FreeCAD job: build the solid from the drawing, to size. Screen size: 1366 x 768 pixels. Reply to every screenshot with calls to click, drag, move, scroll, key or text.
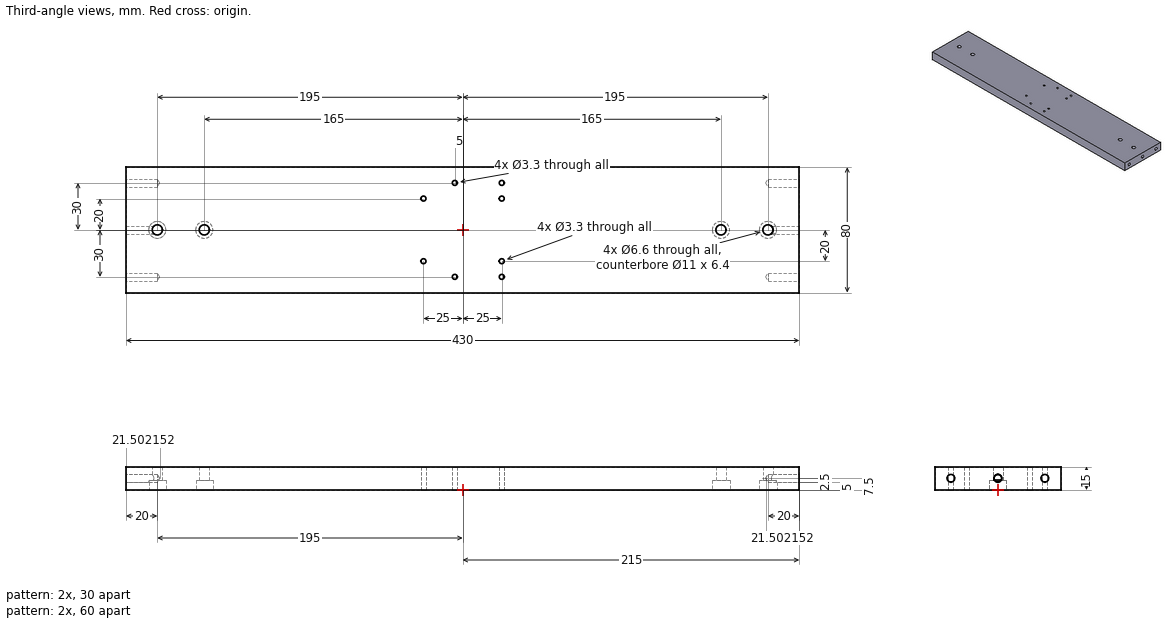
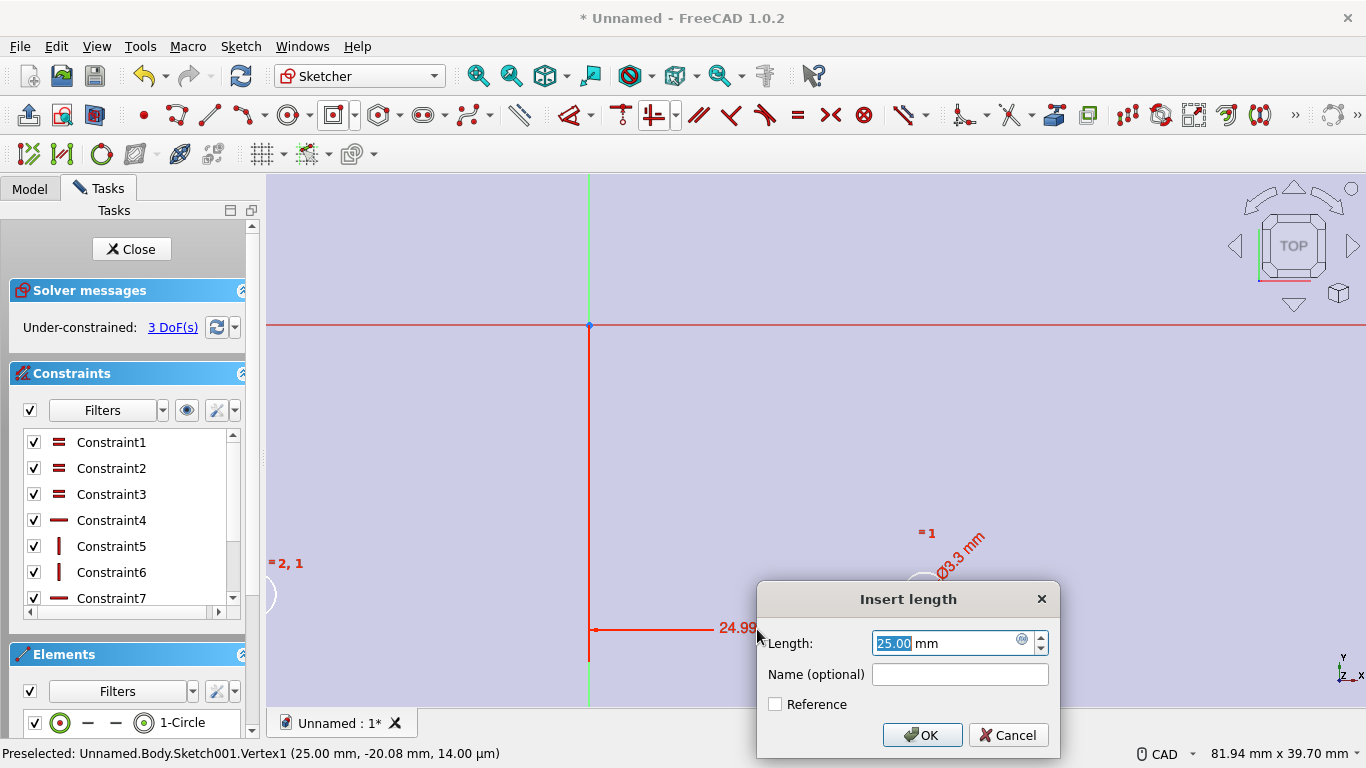
text(25)
key(Return)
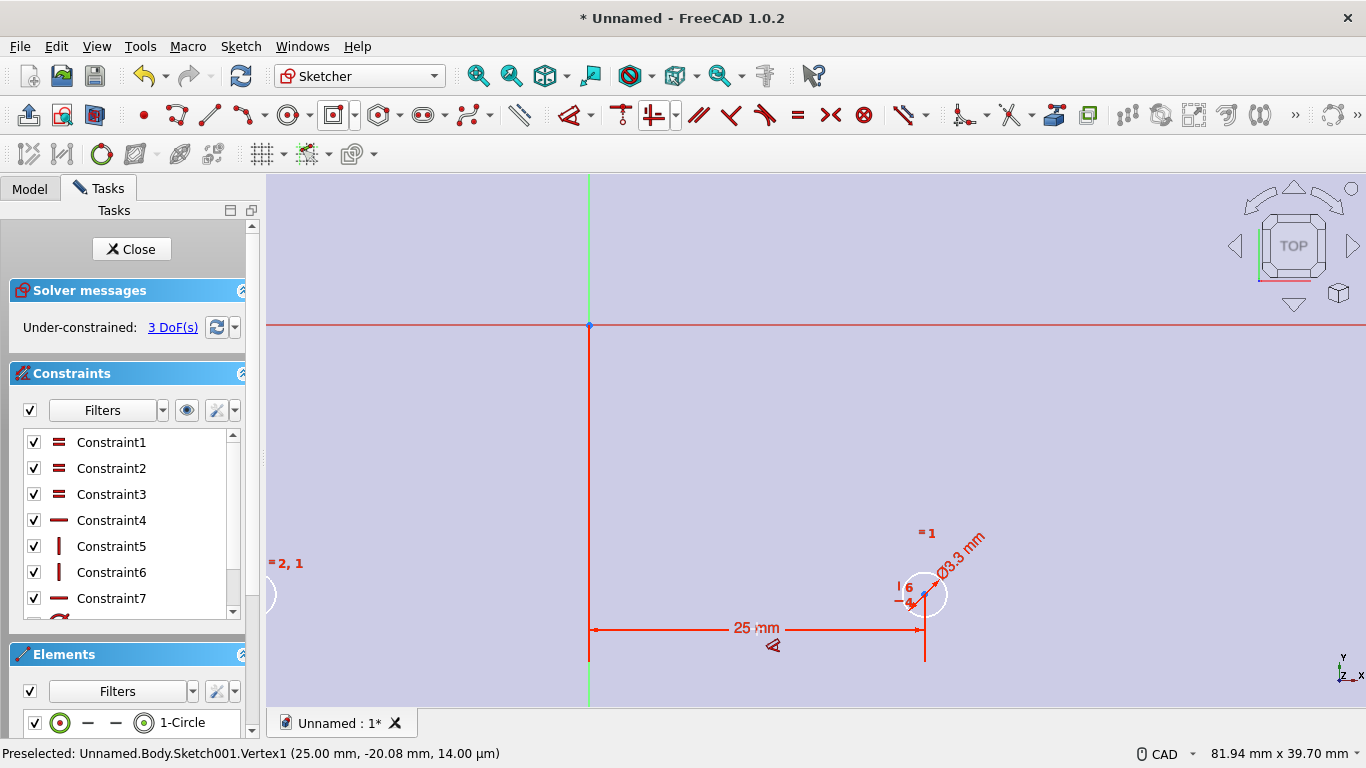
click(925, 595)
click(959, 460)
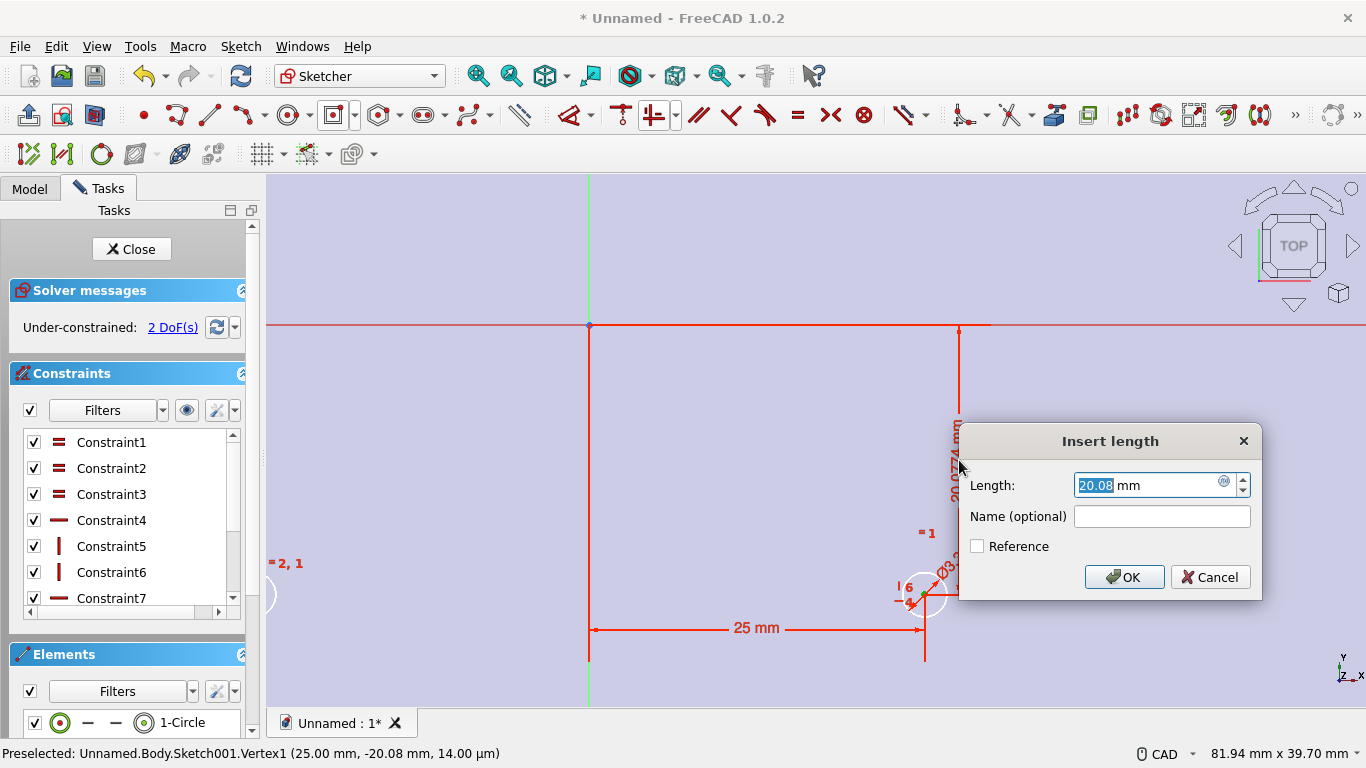
text(20)
key(Return)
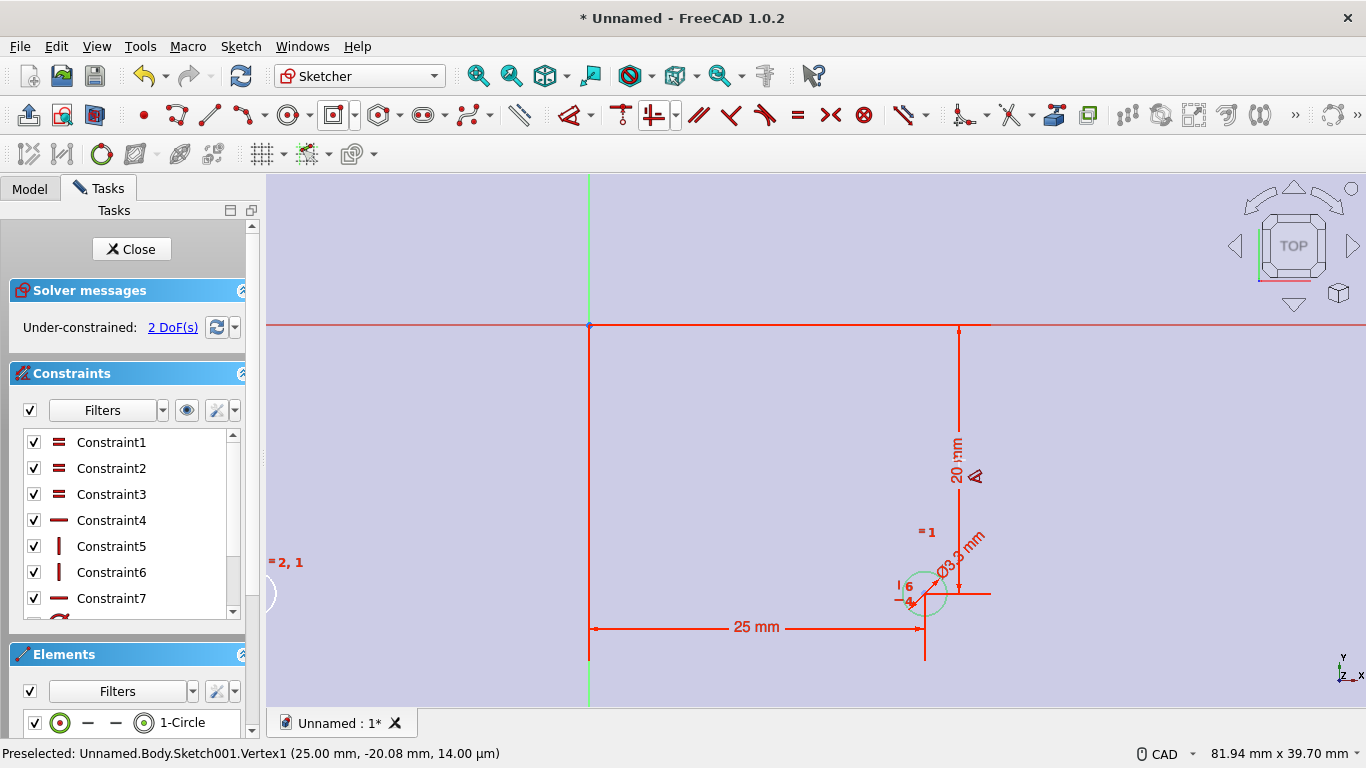
scroll(940, 581, down, 3)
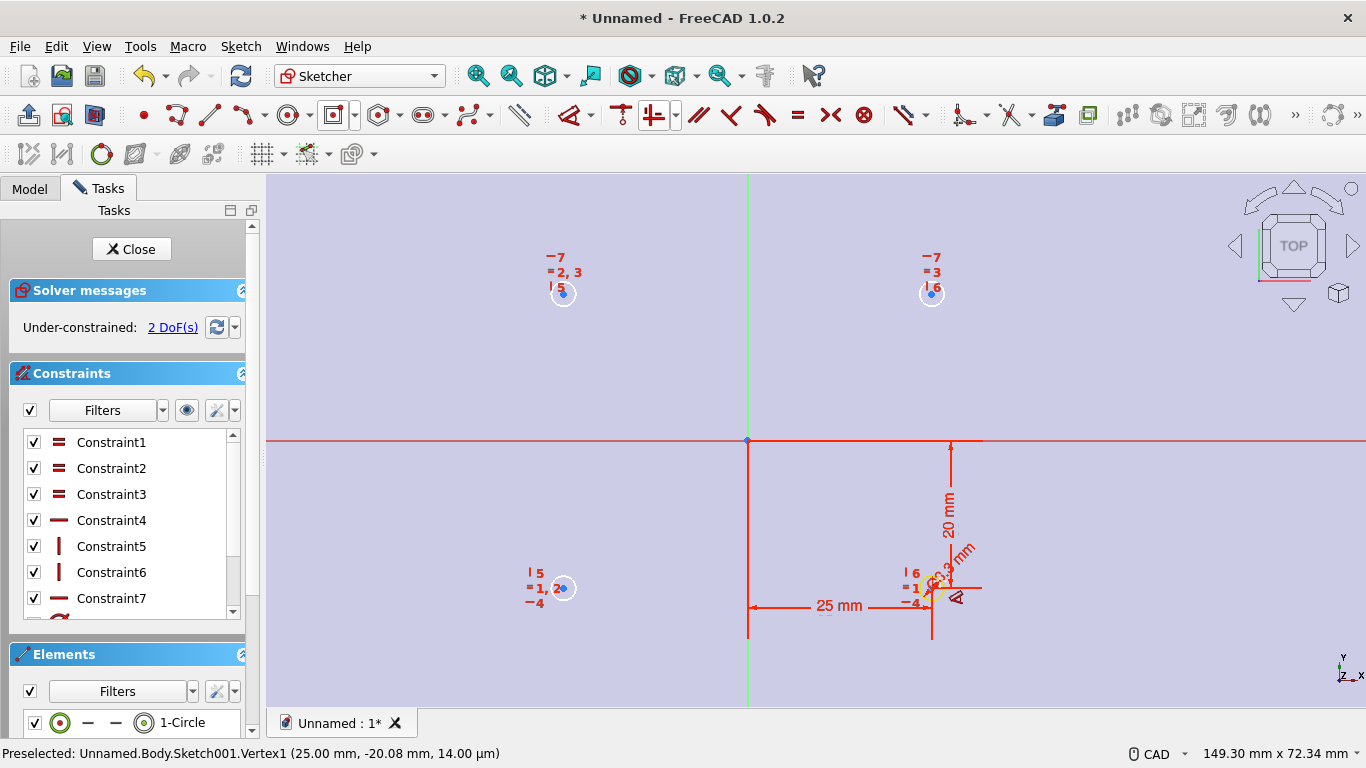
click(564, 588)
click(656, 622)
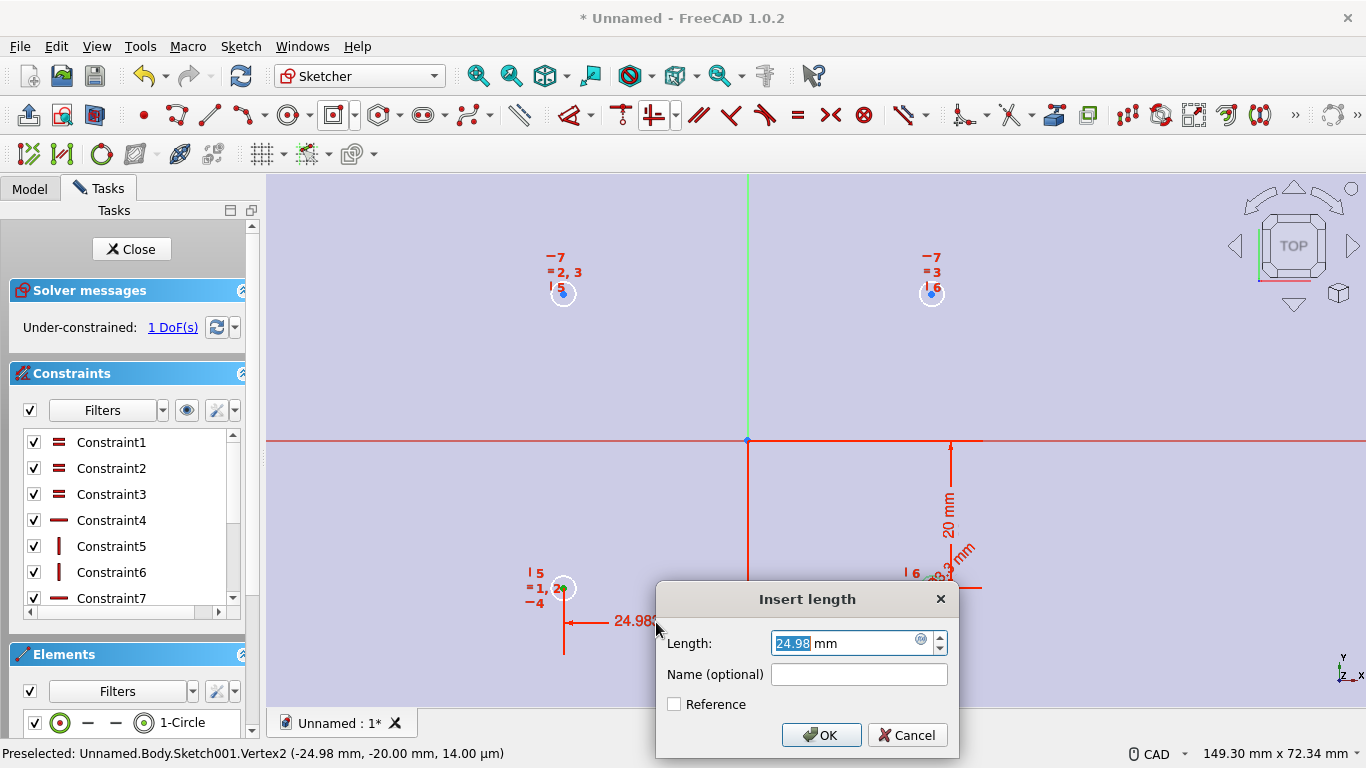
text(25)
key(Return)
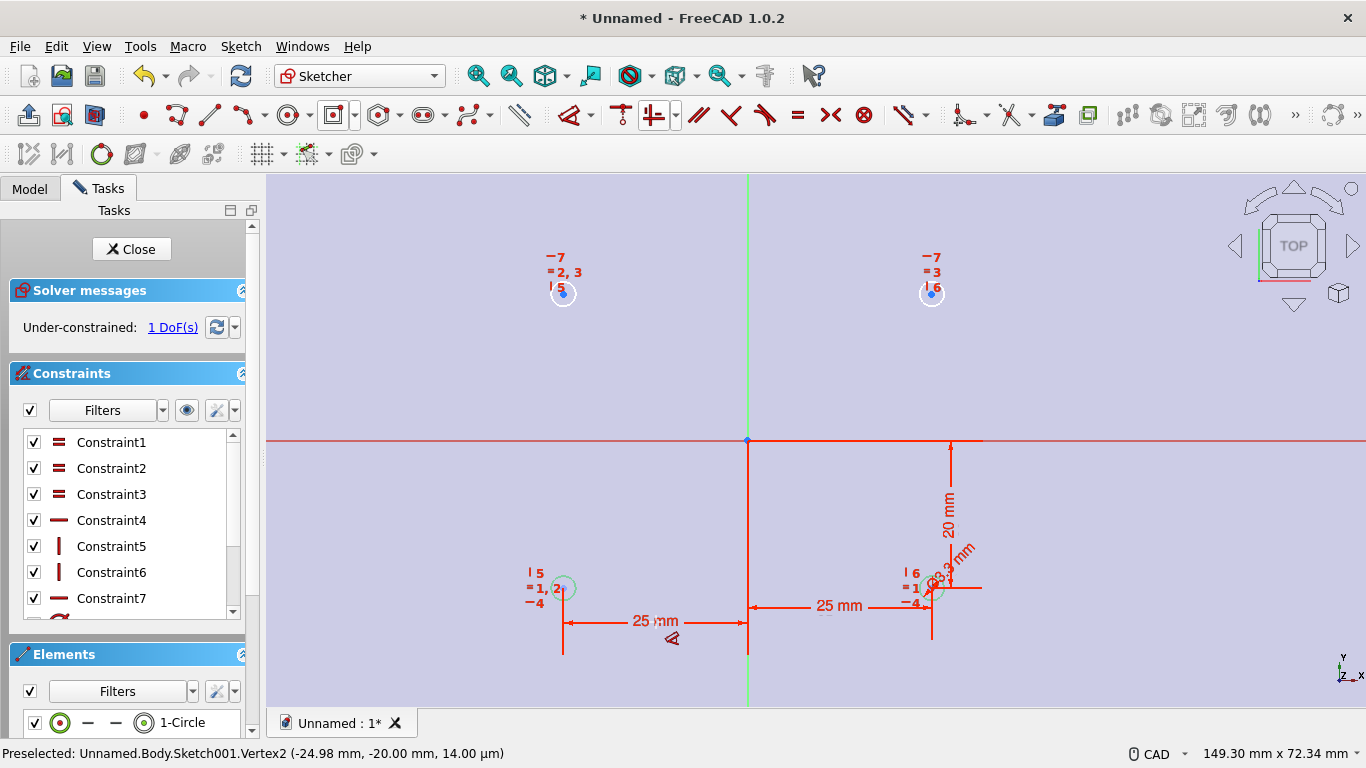
click(563, 294)
click(529, 367)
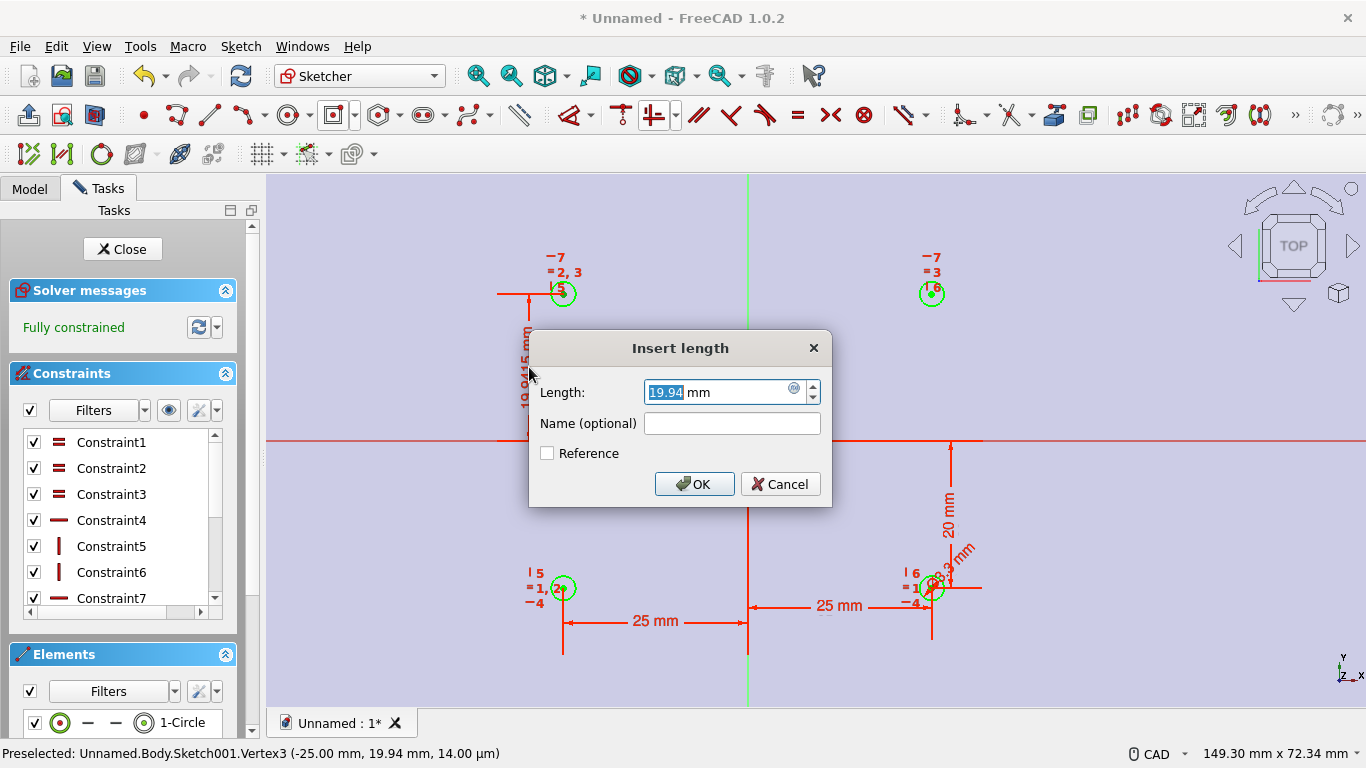
text(20)
key(Return)
key(Escape)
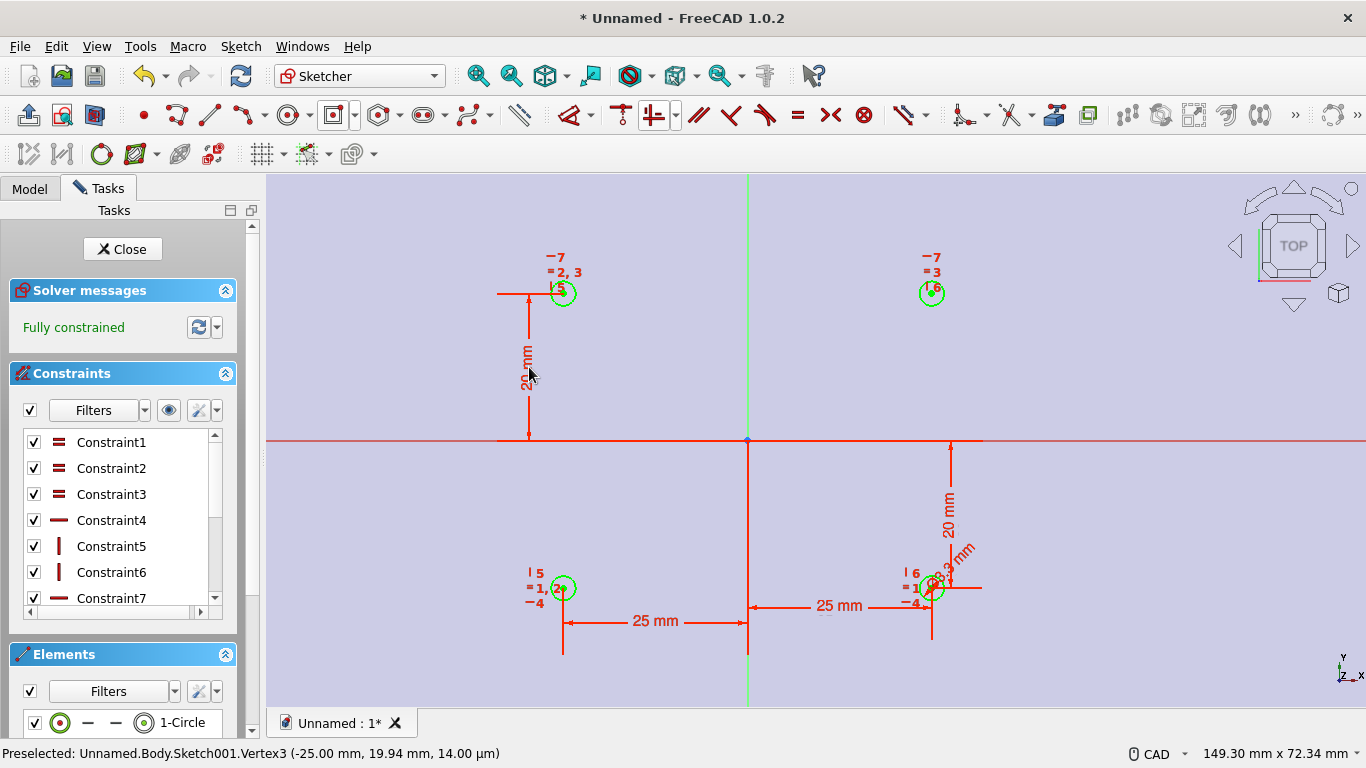
click(123, 249)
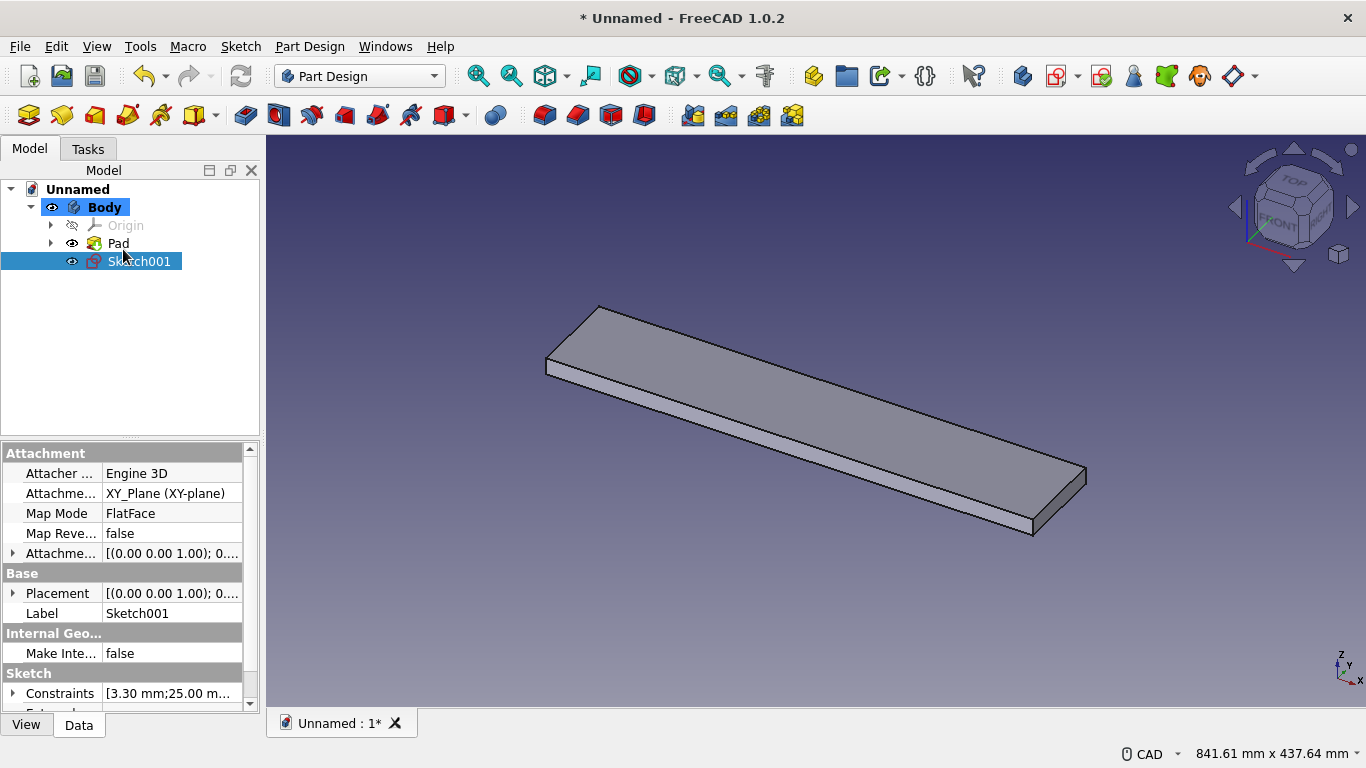
click(279, 116)